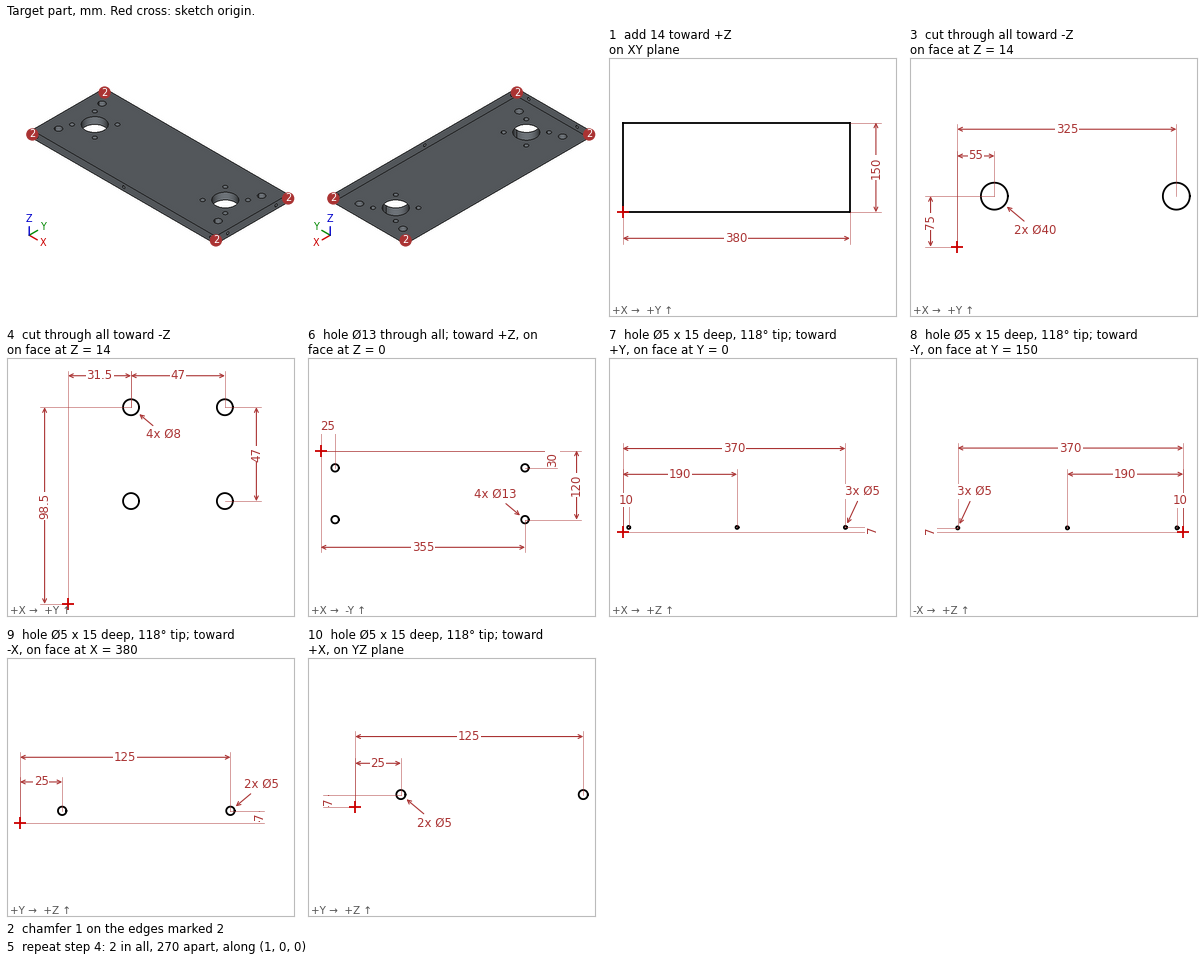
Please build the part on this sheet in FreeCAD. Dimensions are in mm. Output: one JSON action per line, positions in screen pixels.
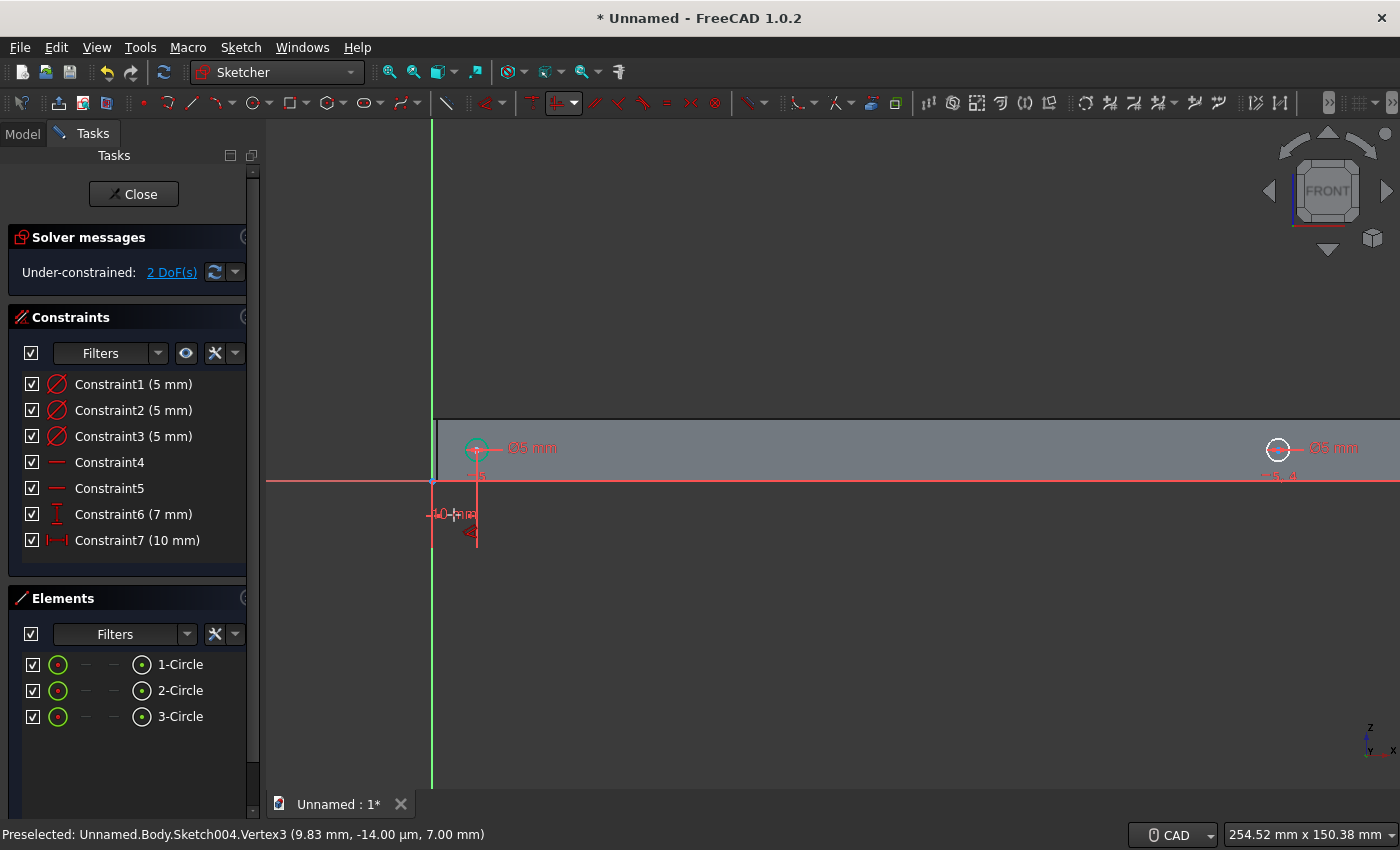
{"action": "scroll", "coordinate": [475, 450], "scroll_direction": "down", "scroll_amount": 5}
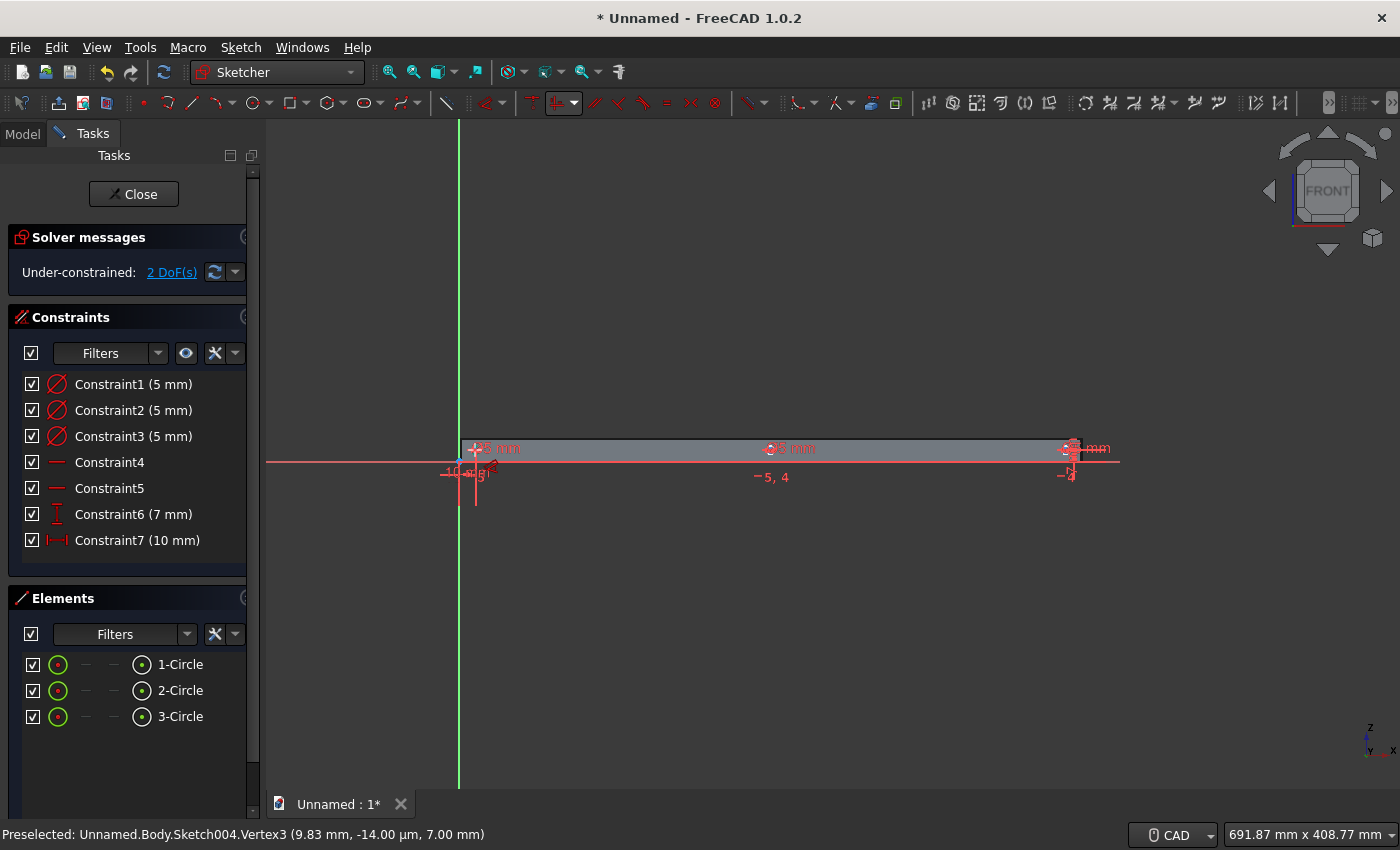
{"action": "left_click", "coordinate": [1066, 450]}
{"action": "left_click", "coordinate": [763, 496]}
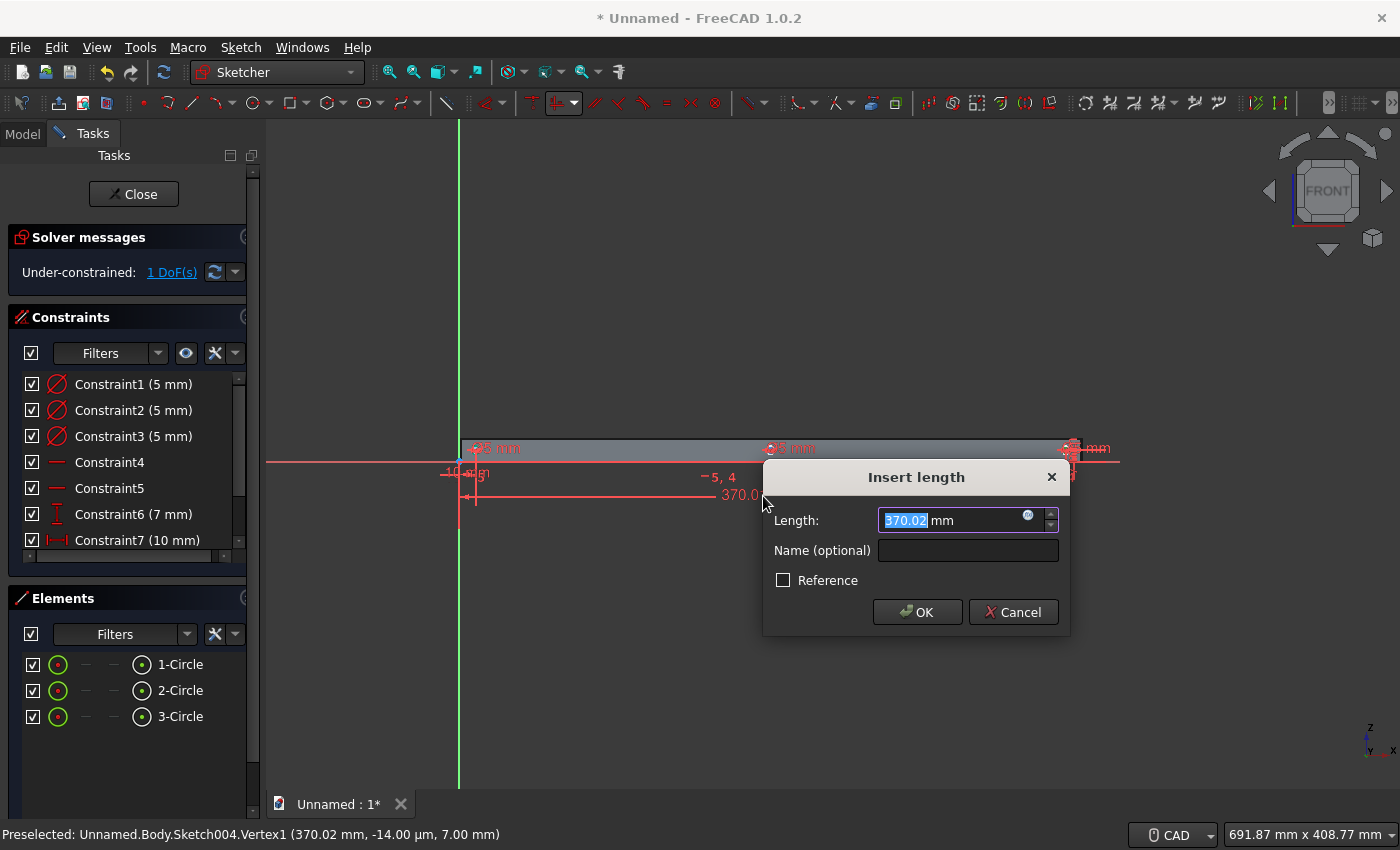
{"action": "type", "text": "370"}
{"action": "key", "text": "Return"}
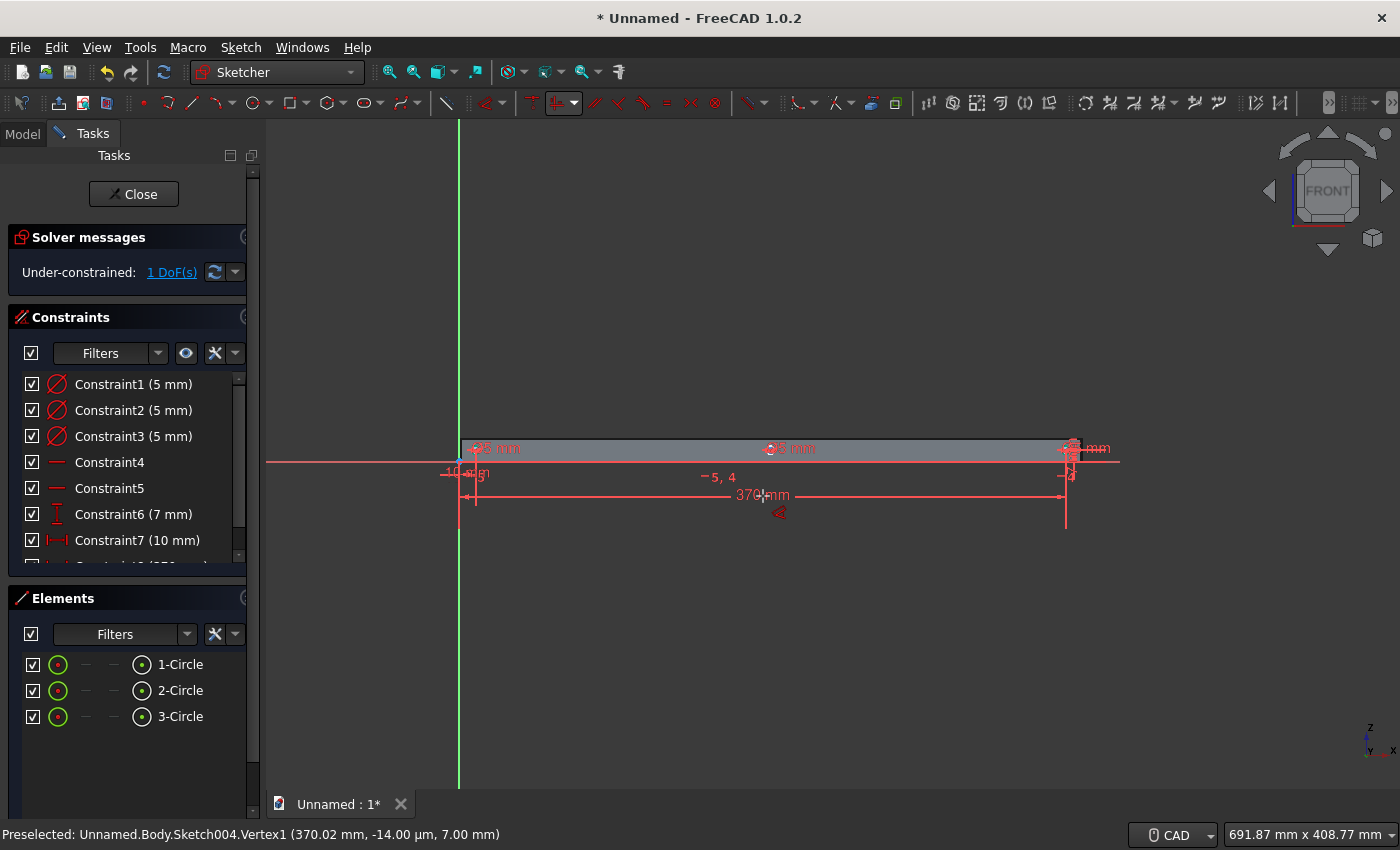
{"action": "left_click", "coordinate": [771, 450]}
{"action": "left_click", "coordinate": [615, 496]}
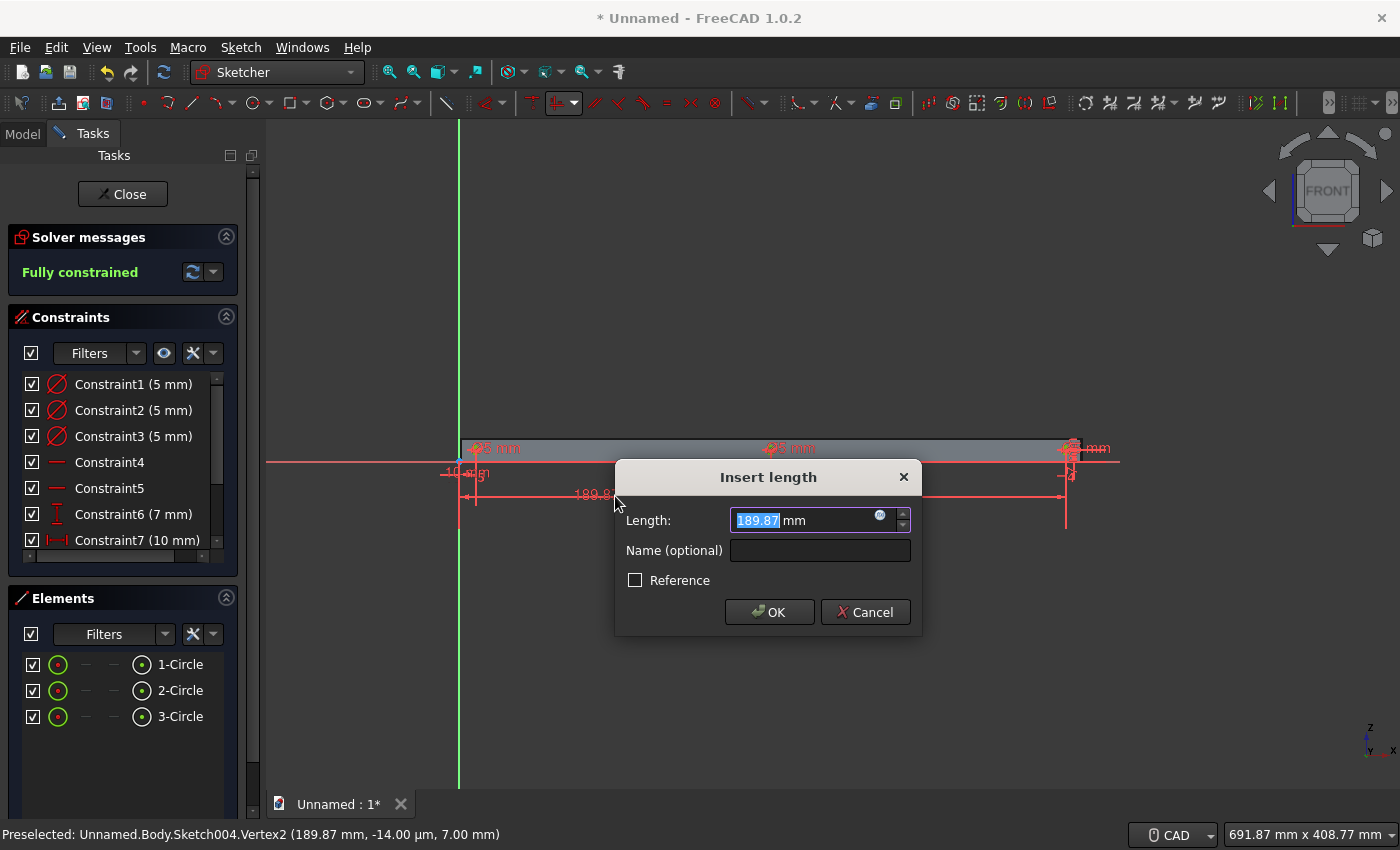
{"action": "type", "text": "190"}
{"action": "key", "text": "Return"}
{"action": "key", "text": "Escape"}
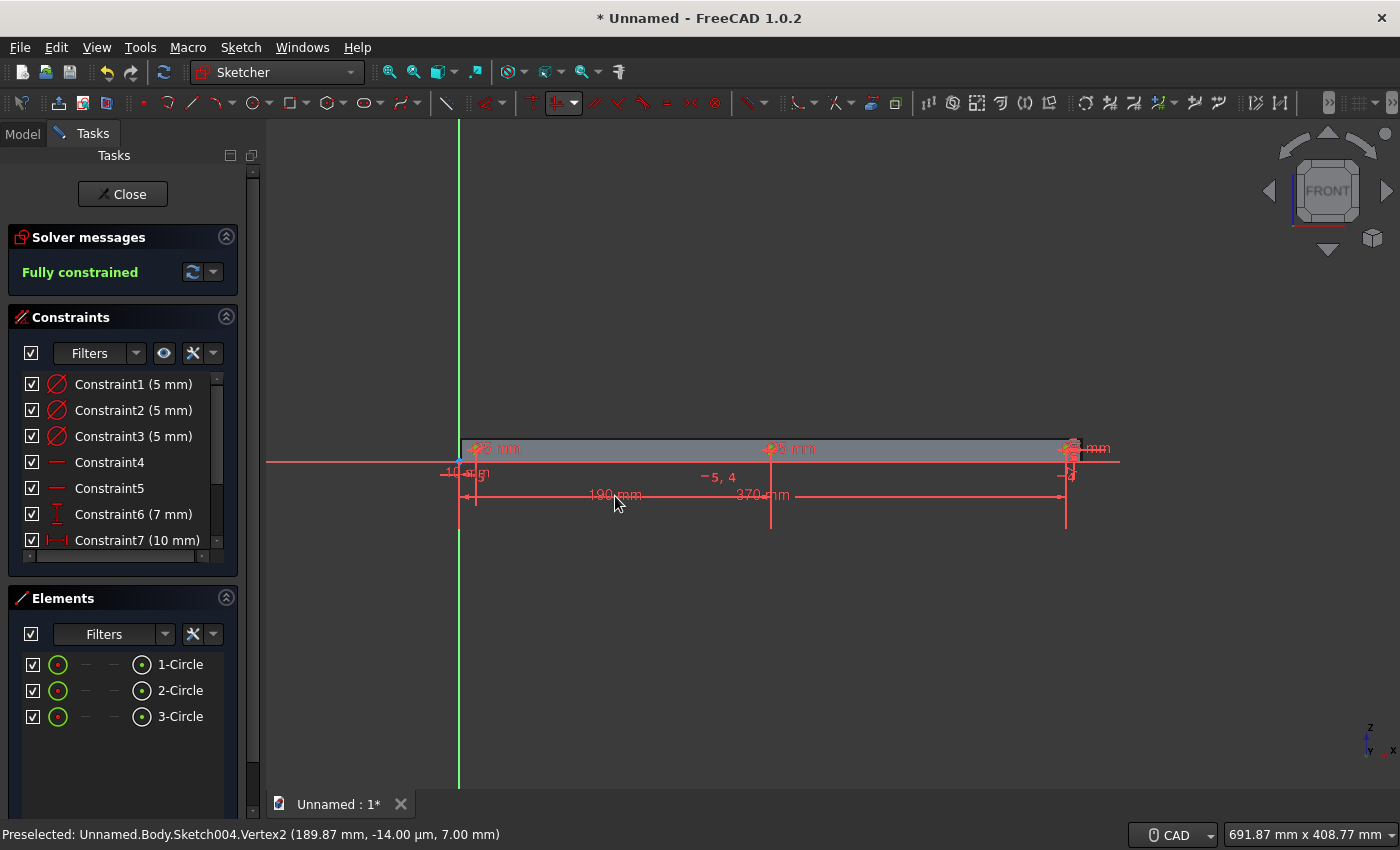
{"action": "left_click", "coordinate": [123, 194]}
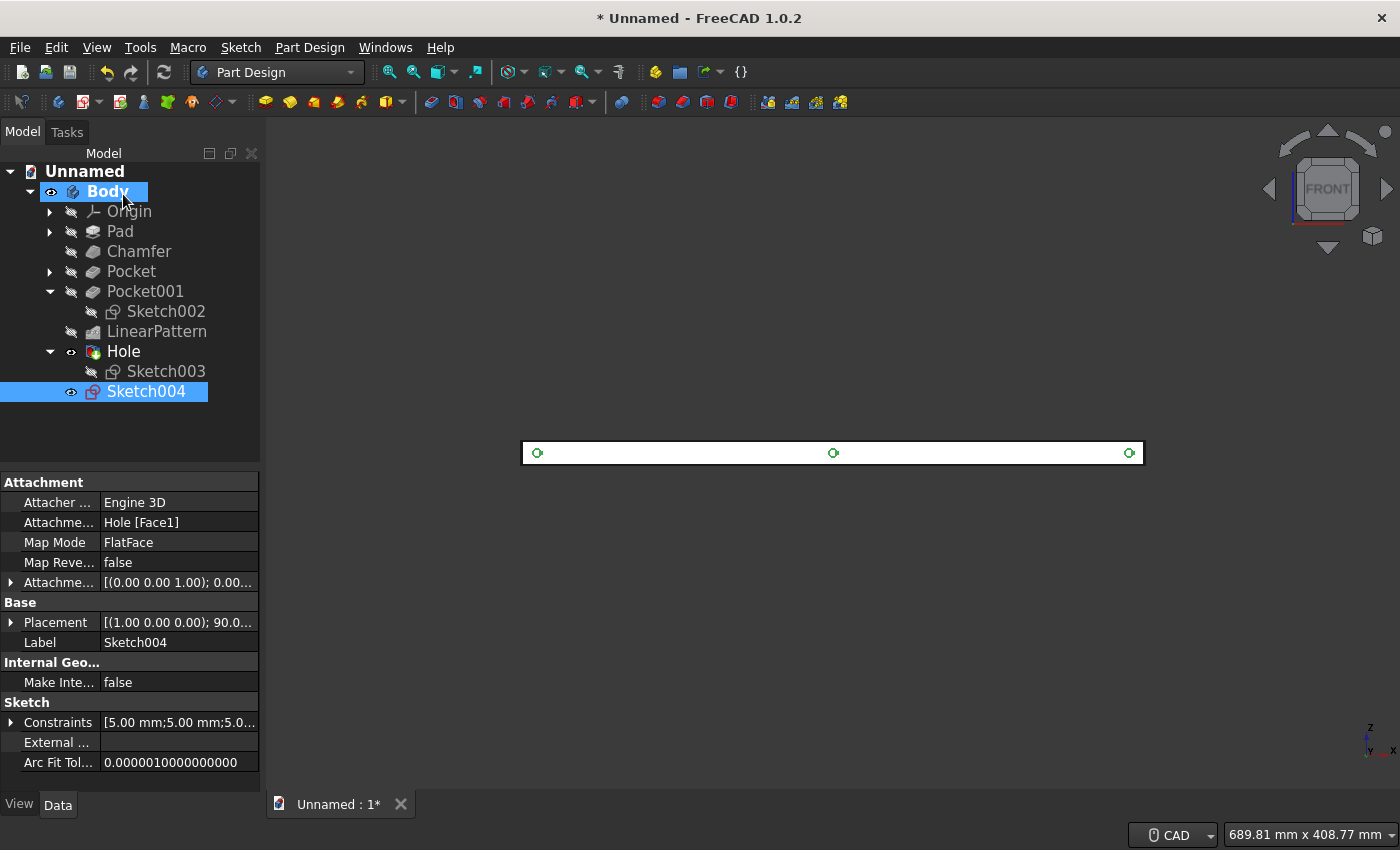
{"action": "left_click", "coordinate": [456, 102]}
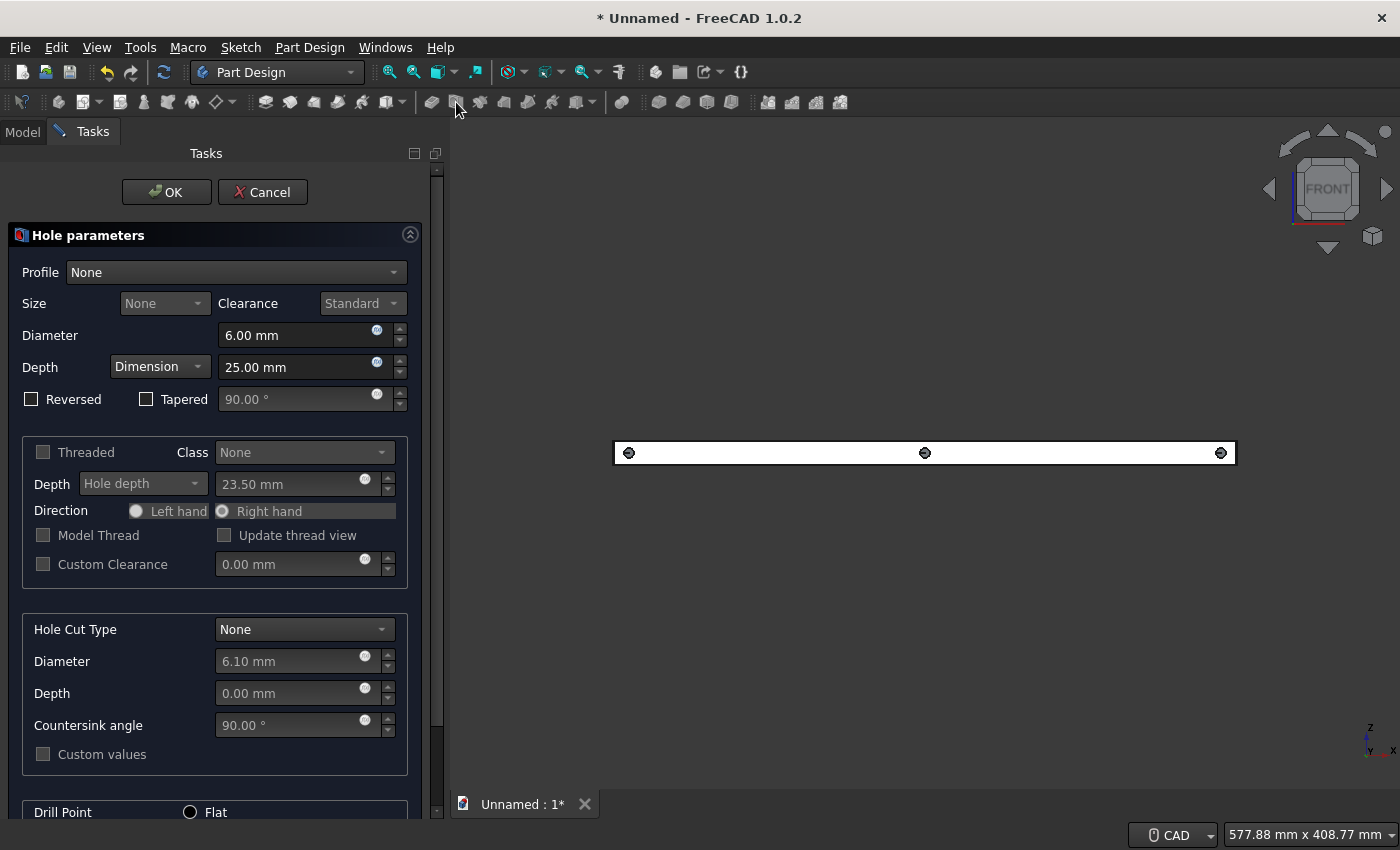
{"action": "triple_click", "coordinate": [305, 335]}